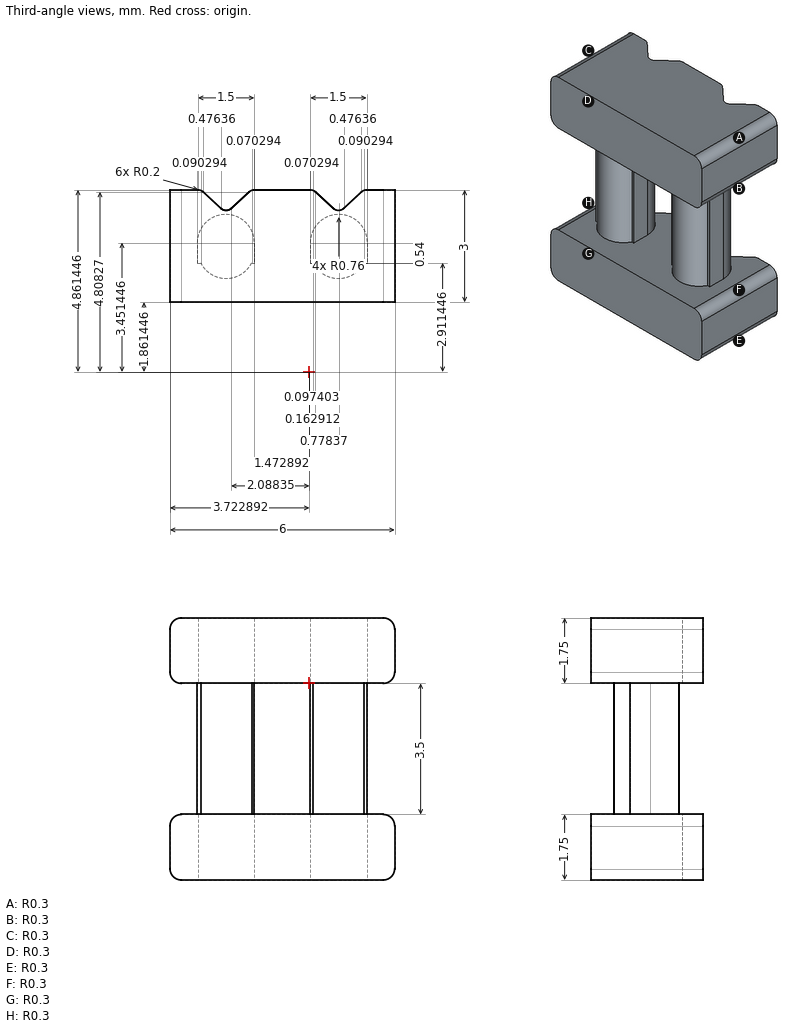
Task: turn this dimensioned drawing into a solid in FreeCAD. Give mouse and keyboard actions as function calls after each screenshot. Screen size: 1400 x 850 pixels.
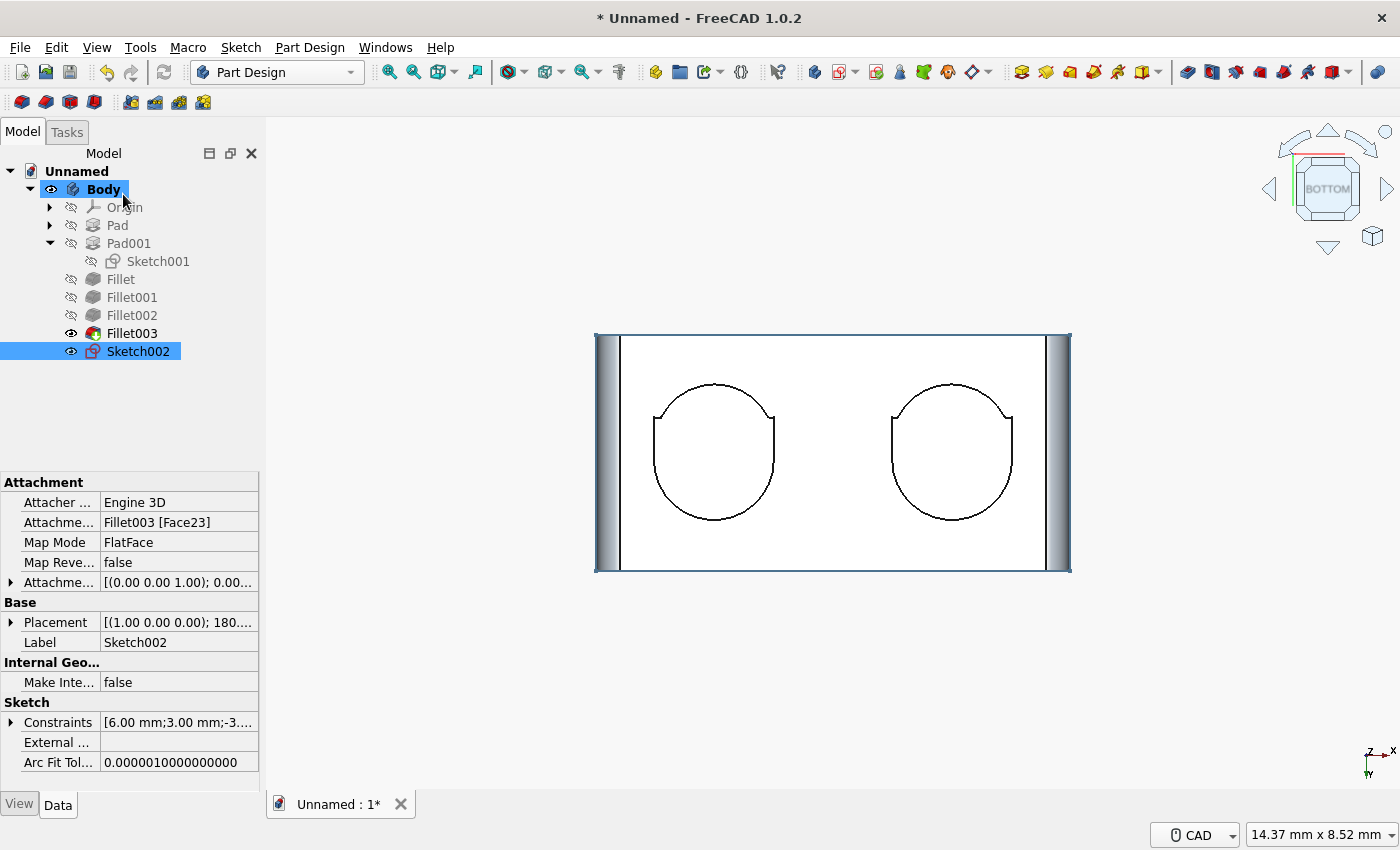
click(1022, 72)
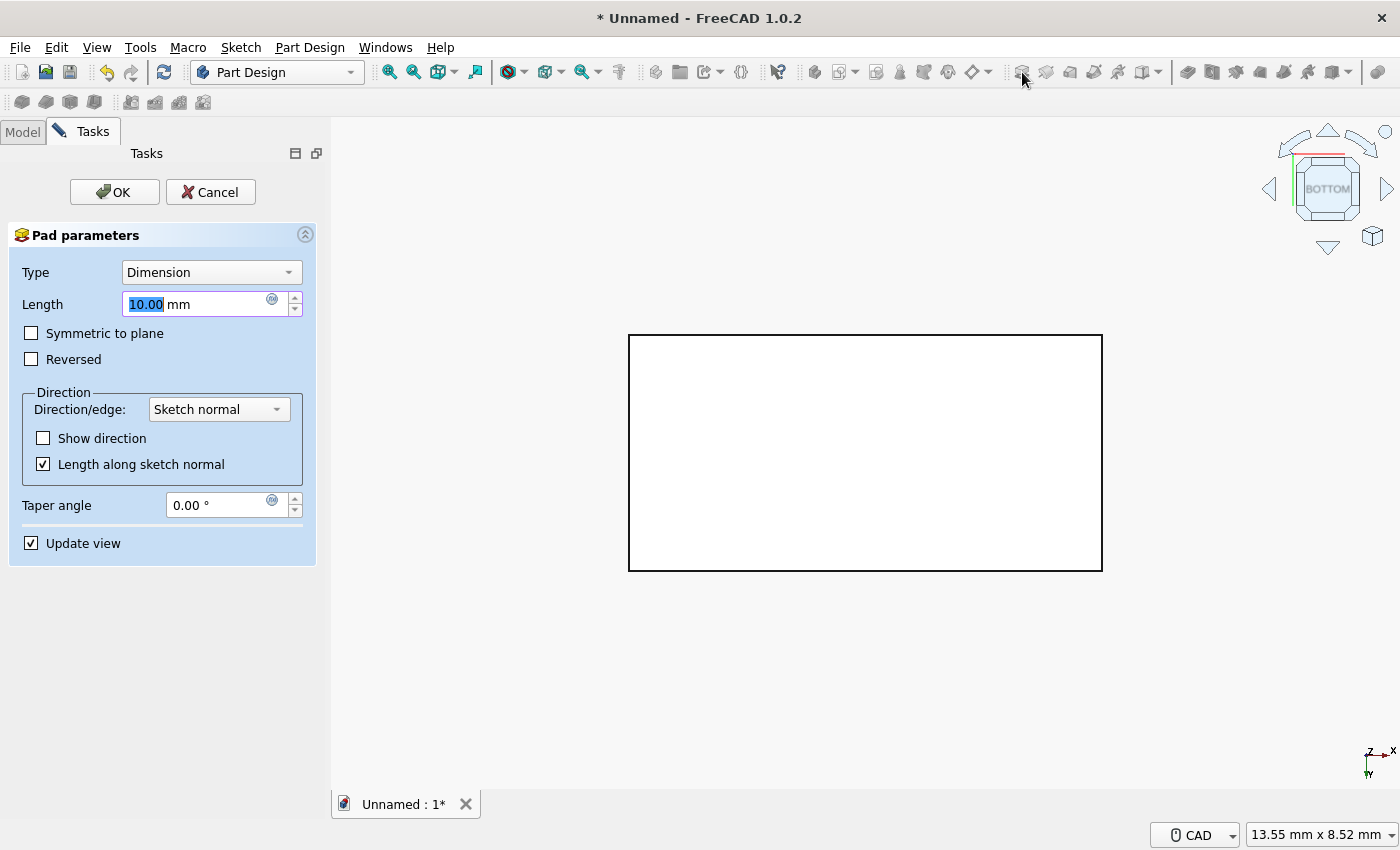
text(1.75)
key(Tab)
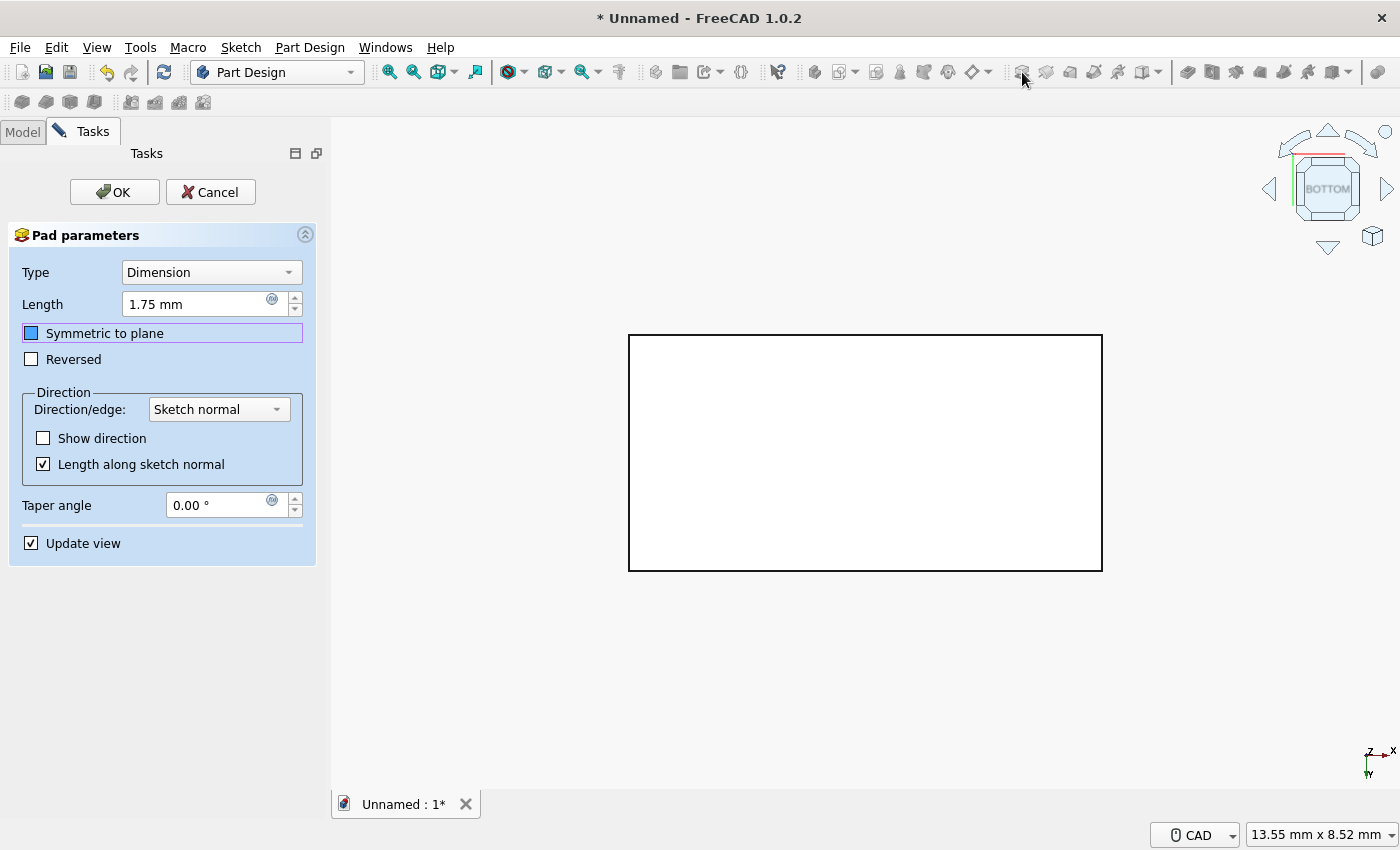
click(115, 192)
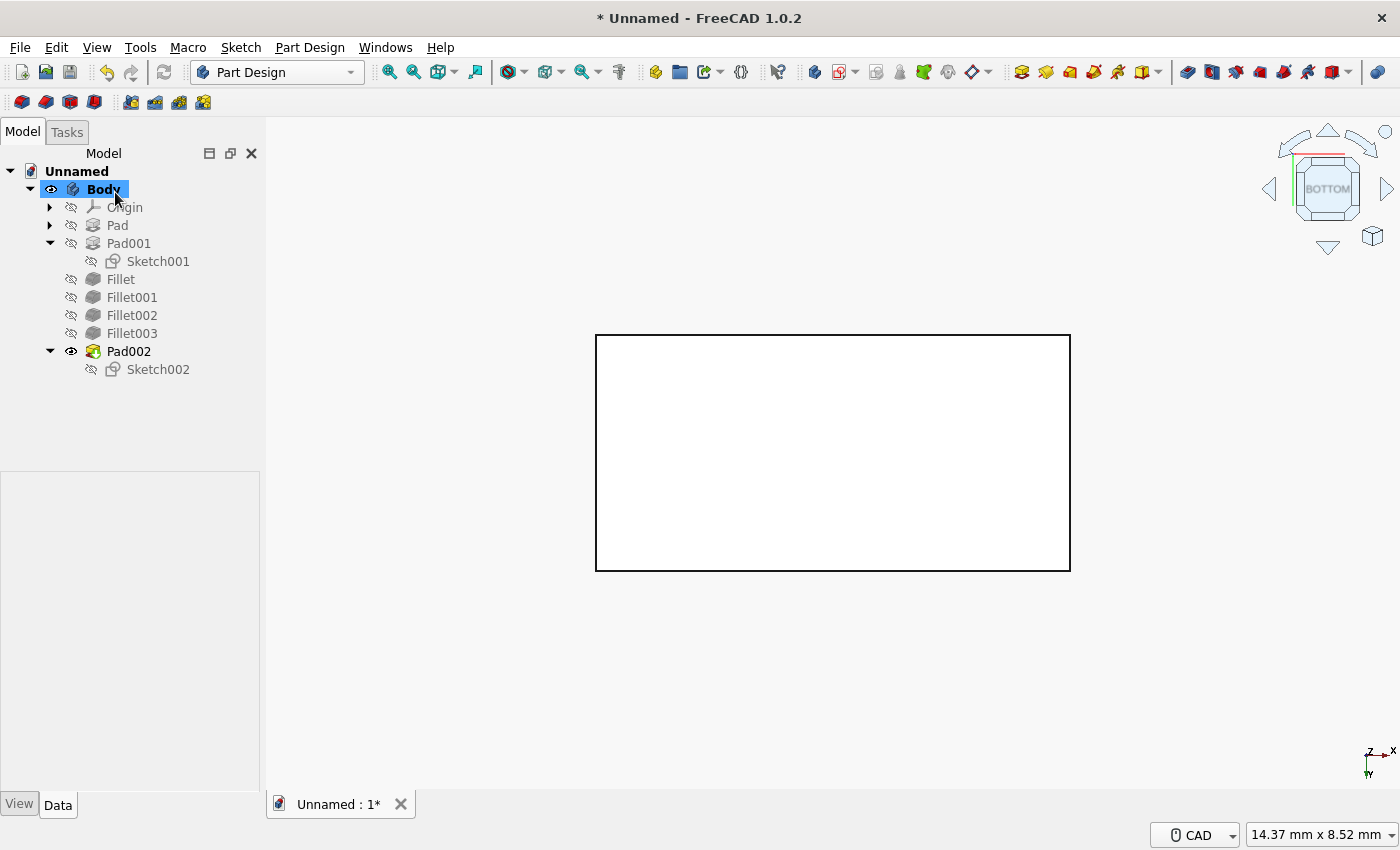
click(390, 72)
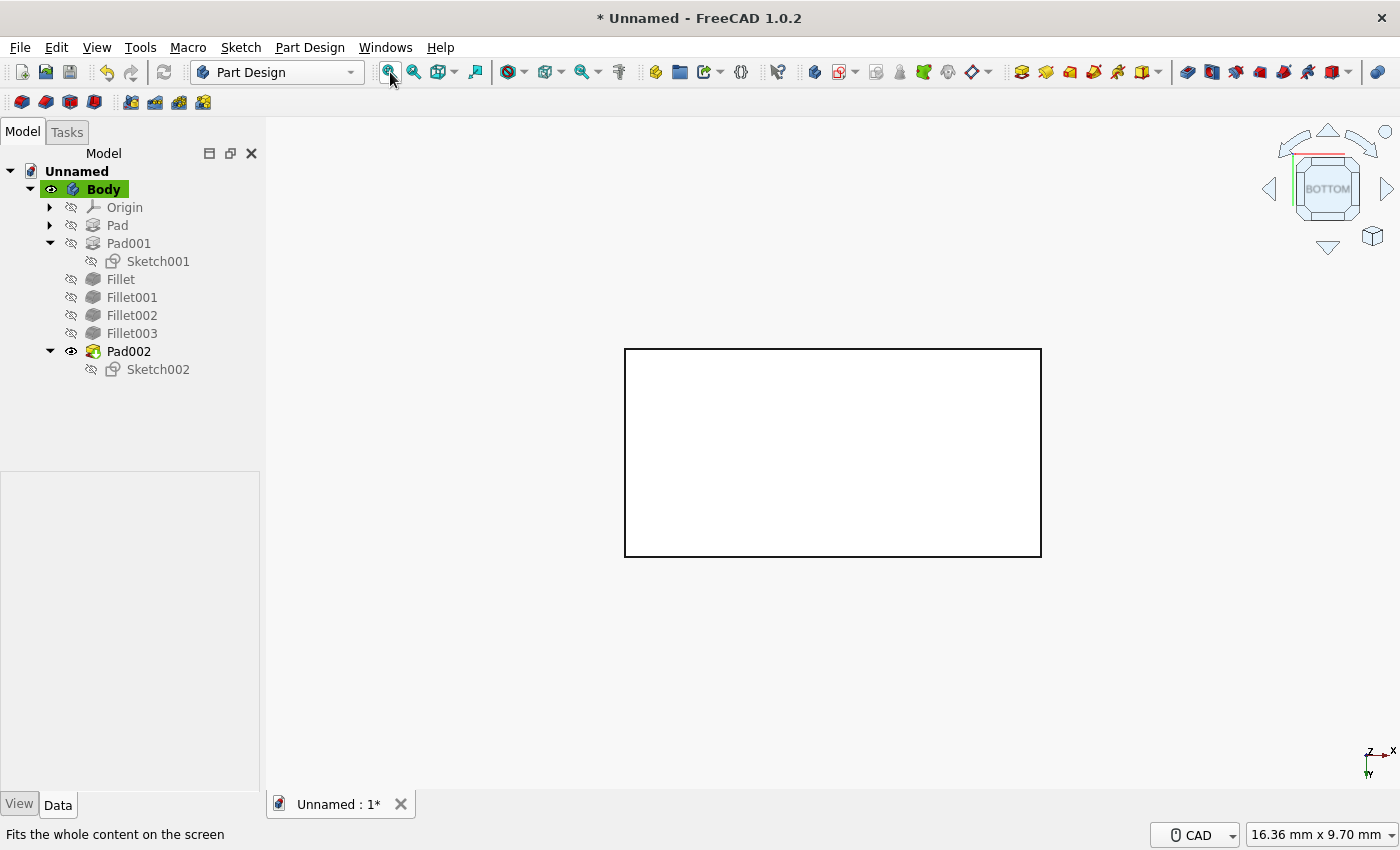
click(1041, 452)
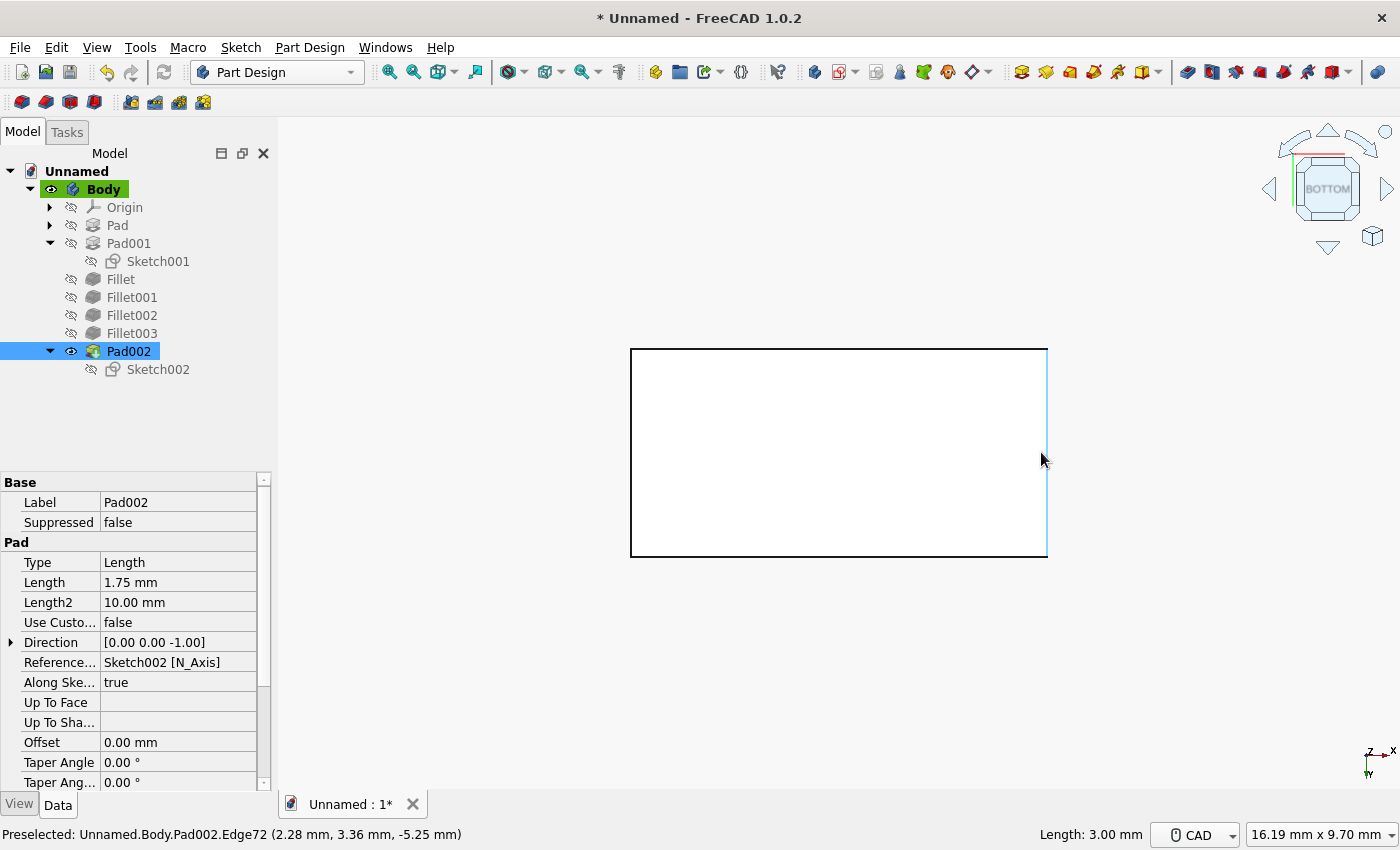
click(22, 102)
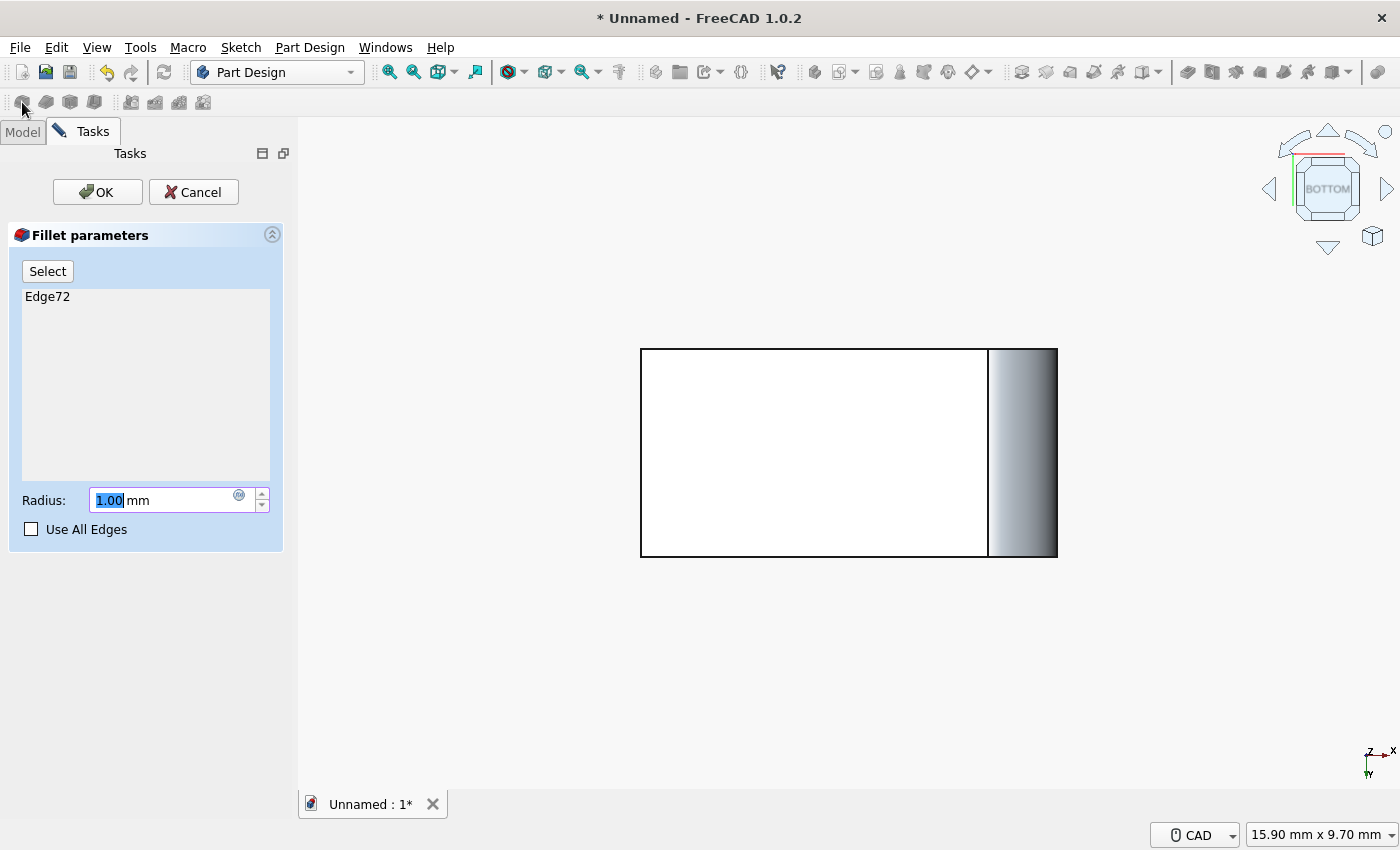
text(0.3)
key(Tab)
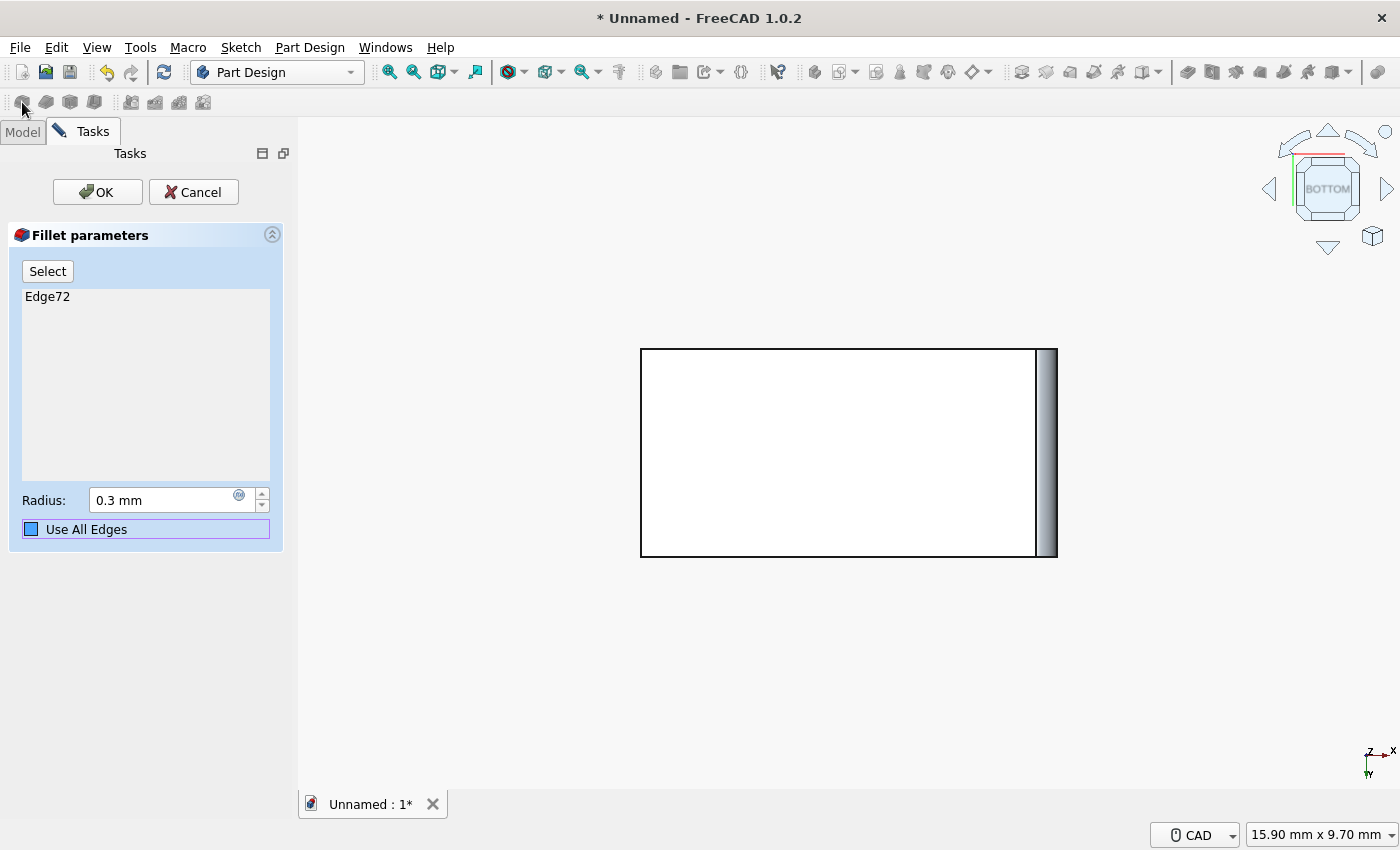
click(98, 192)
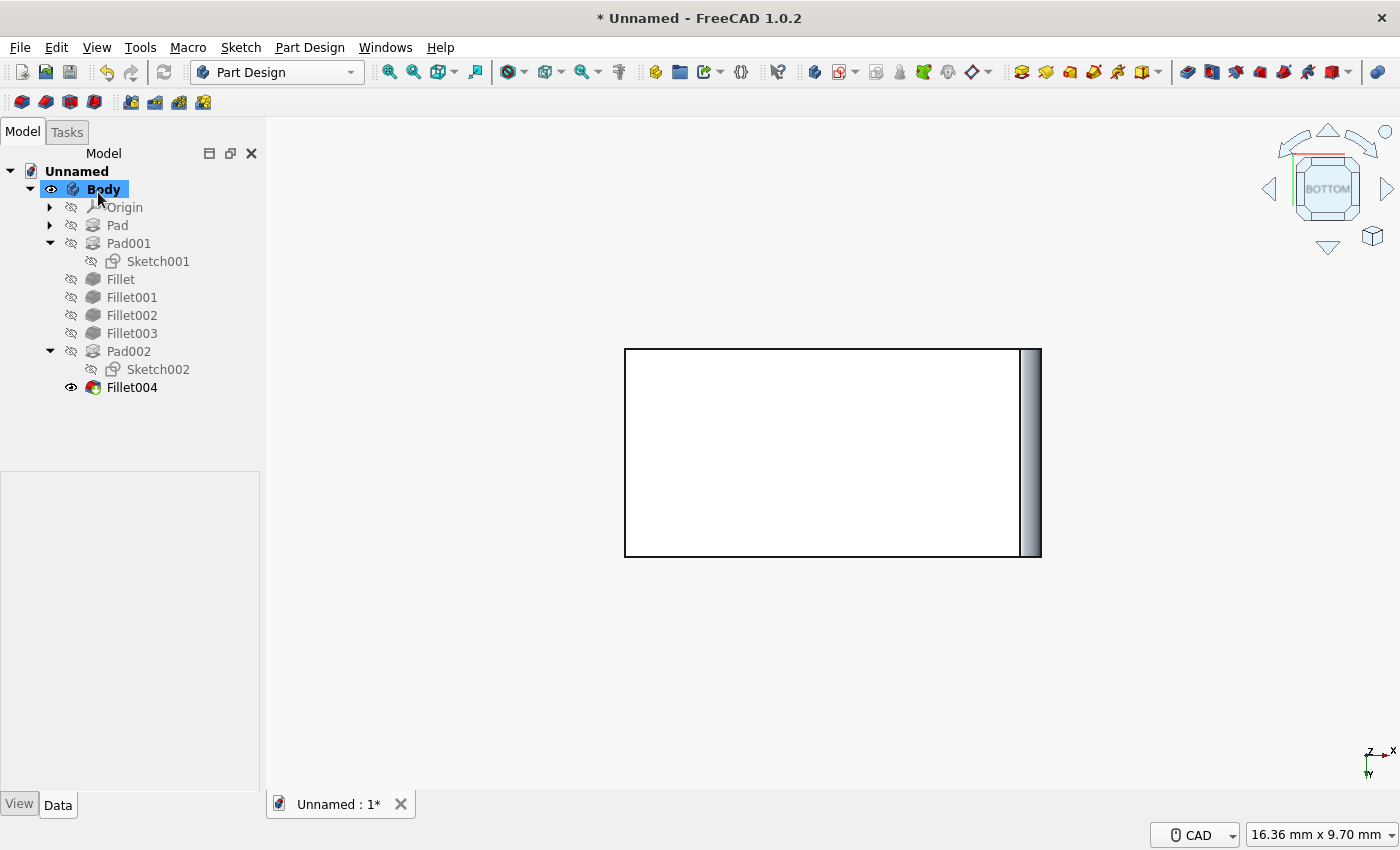
click(390, 72)